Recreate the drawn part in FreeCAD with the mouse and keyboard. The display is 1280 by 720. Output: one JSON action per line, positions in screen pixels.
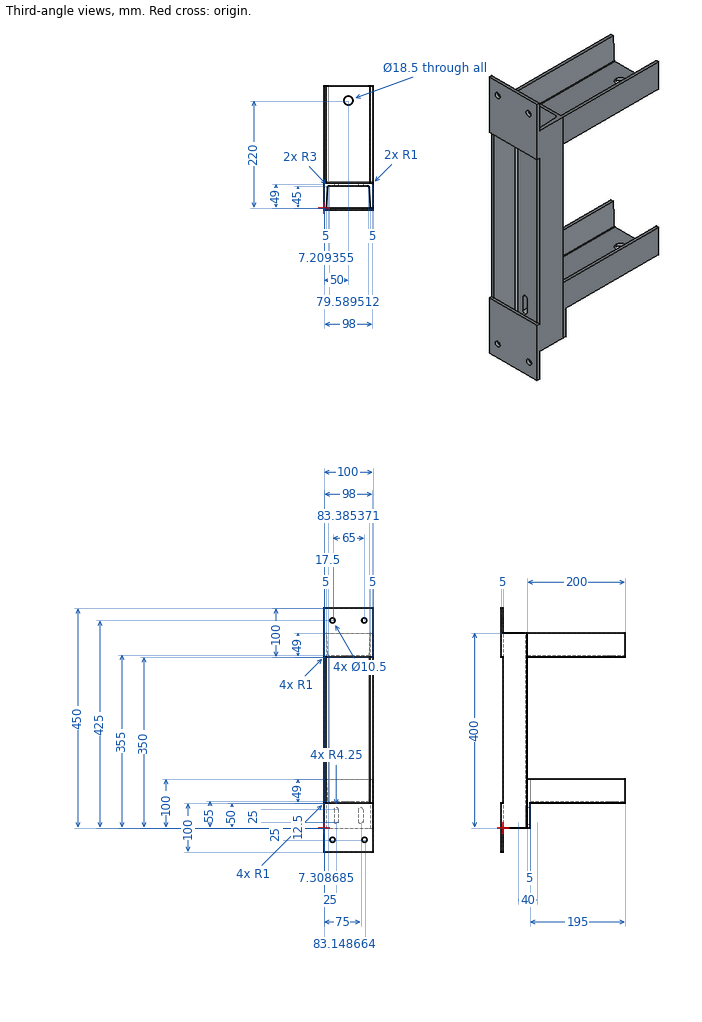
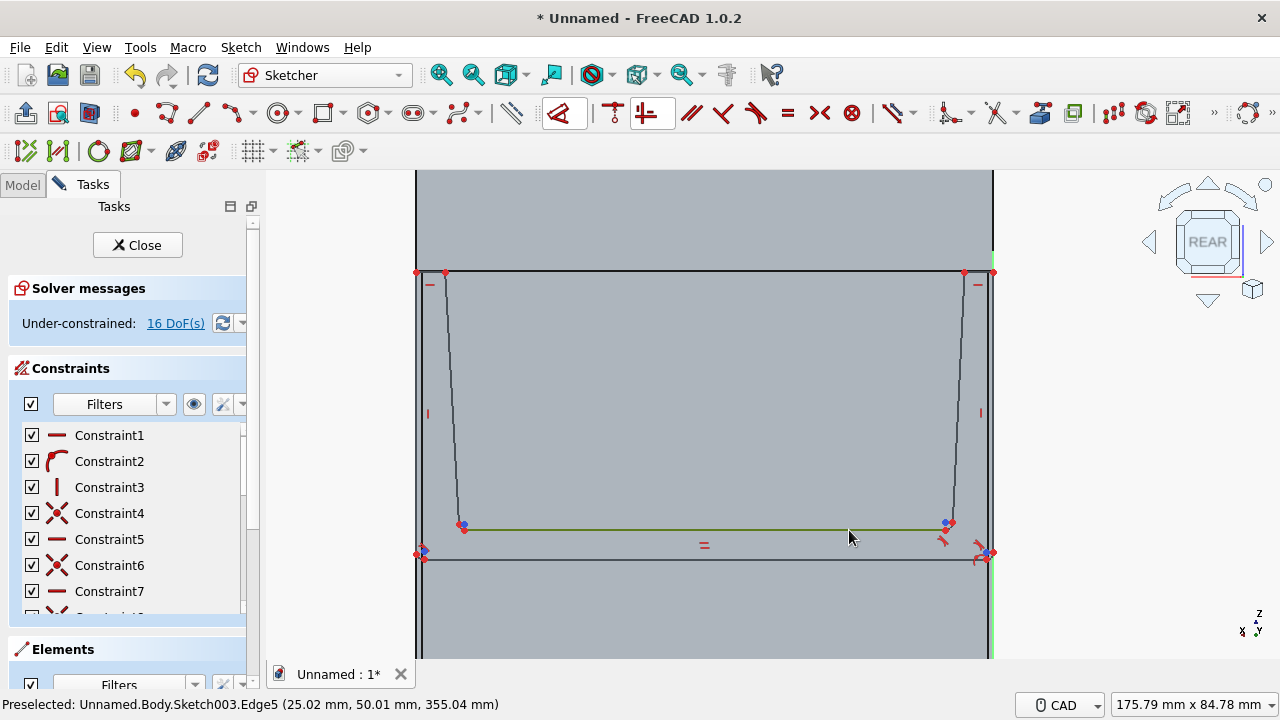
{"action": "scroll", "coordinate": [461, 528], "scroll_direction": "up", "scroll_amount": 7}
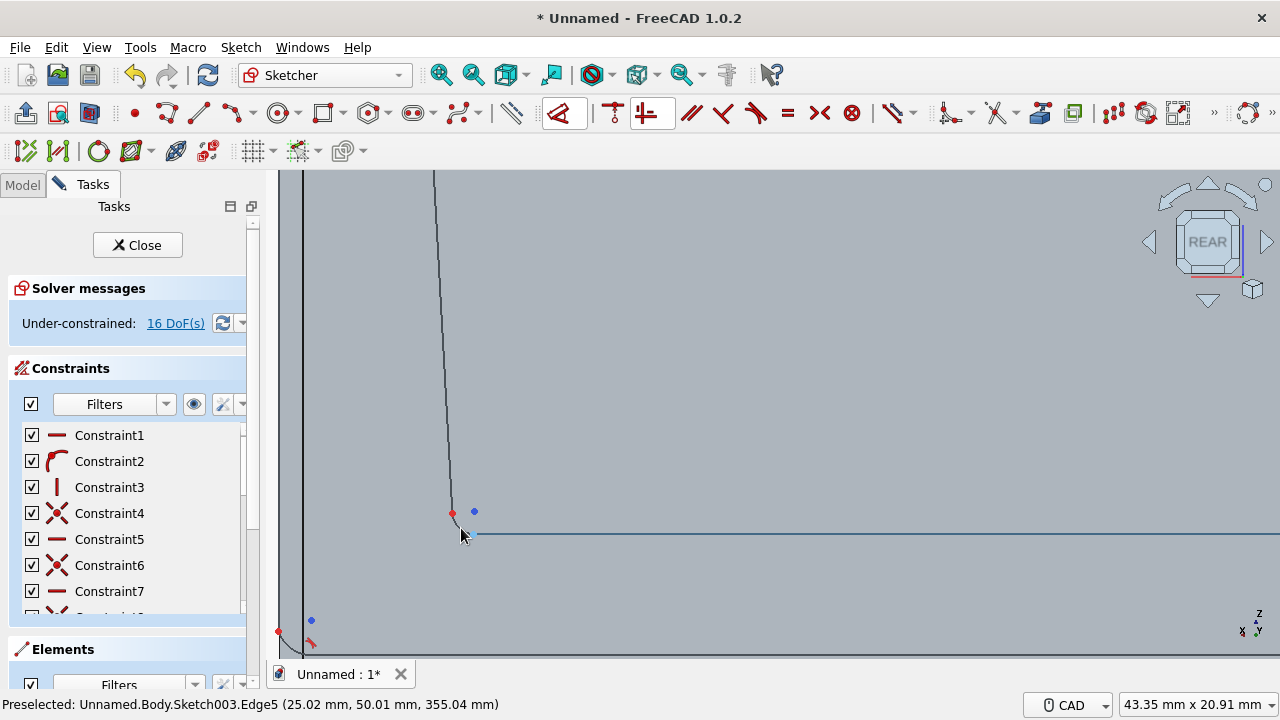
{"action": "left_click", "coordinate": [459, 528]}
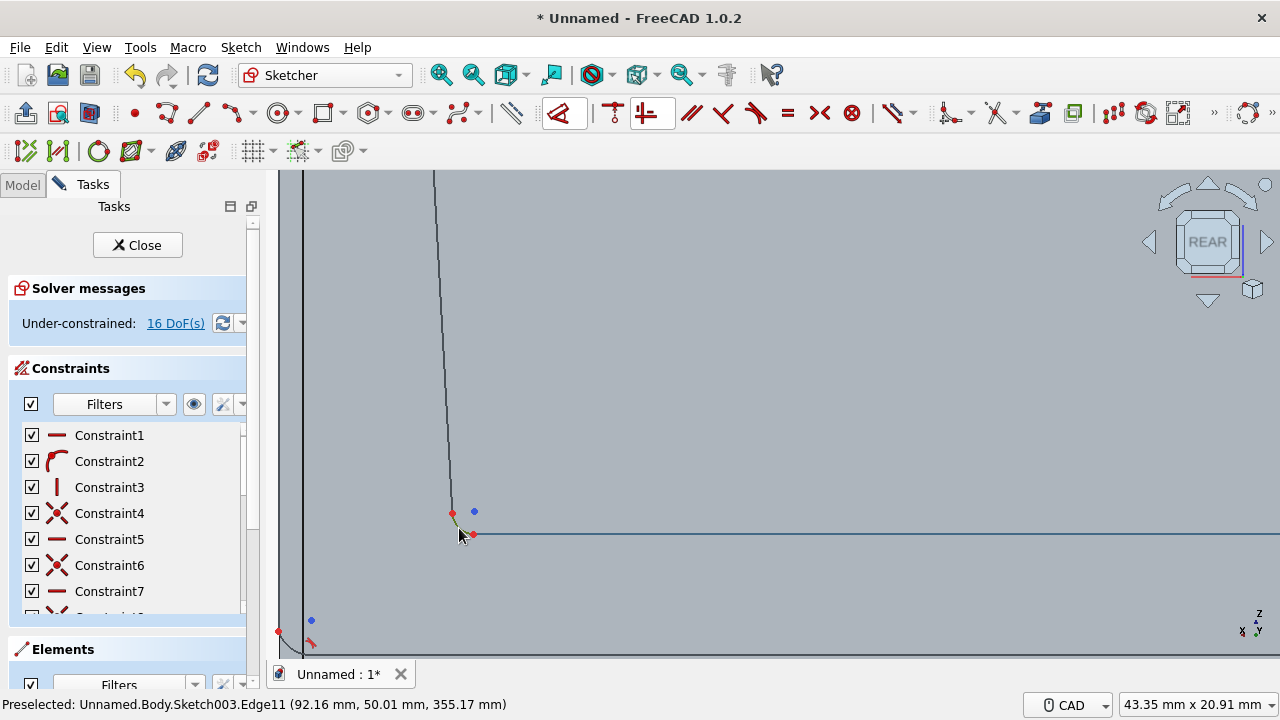
{"action": "left_click", "coordinate": [756, 114]}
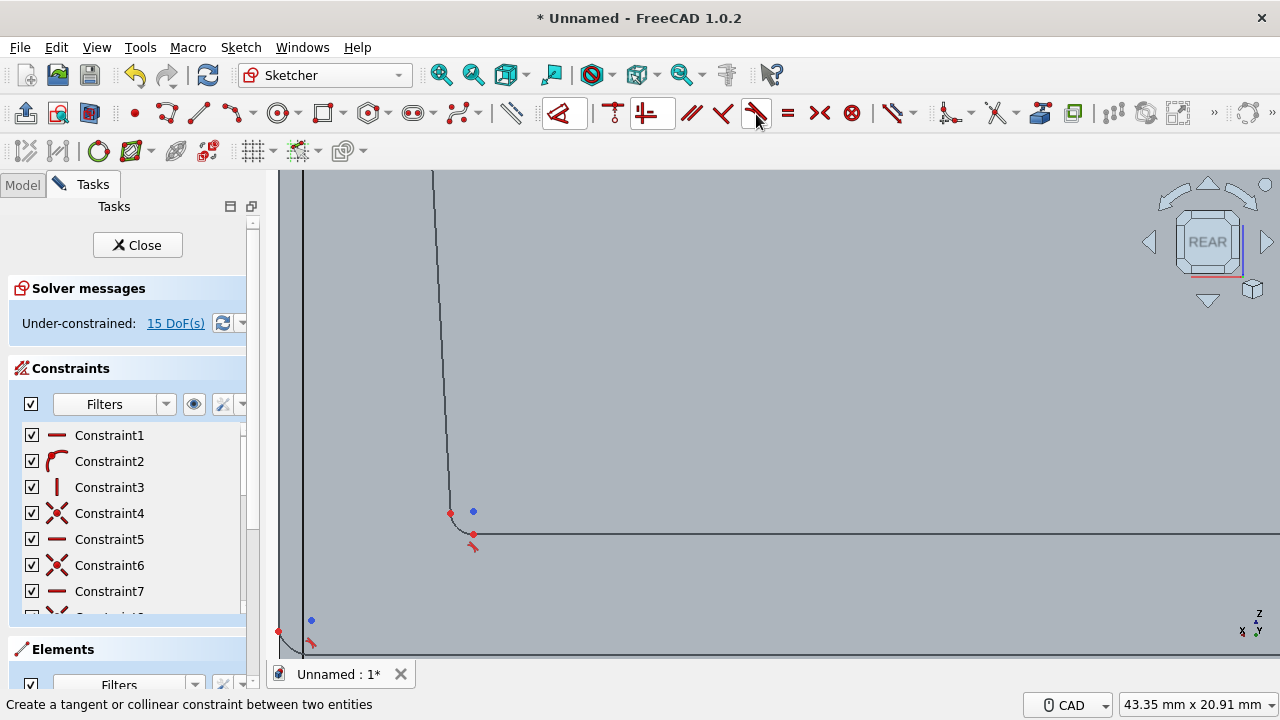
{"action": "scroll", "coordinate": [461, 528], "scroll_direction": "down", "scroll_amount": 7}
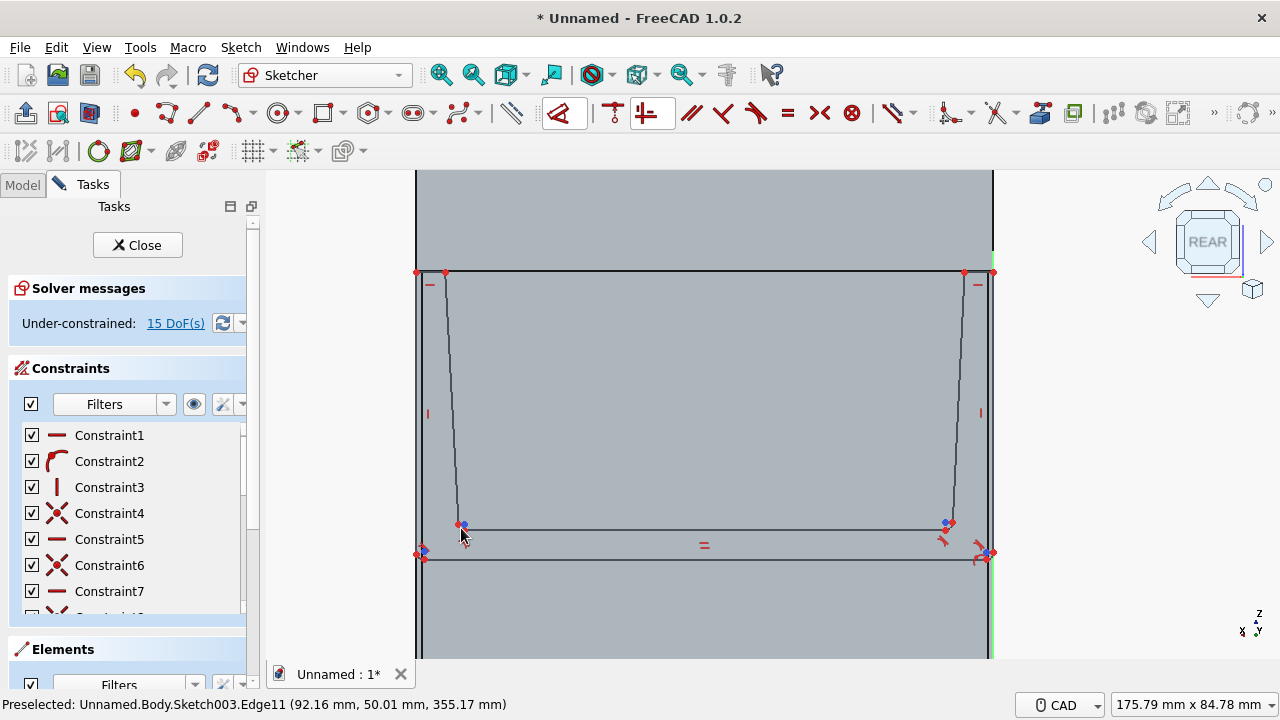
{"action": "left_click", "coordinate": [455, 449]}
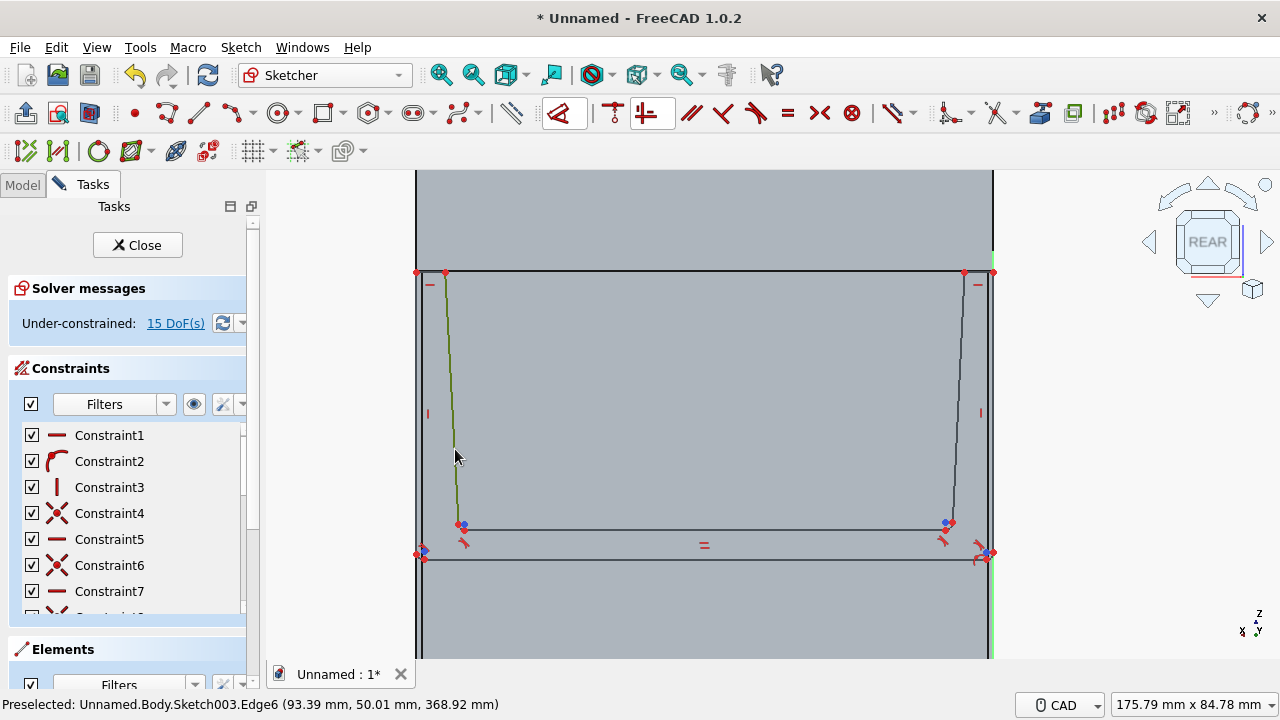
{"action": "scroll", "coordinate": [460, 529], "scroll_direction": "up", "scroll_amount": 7}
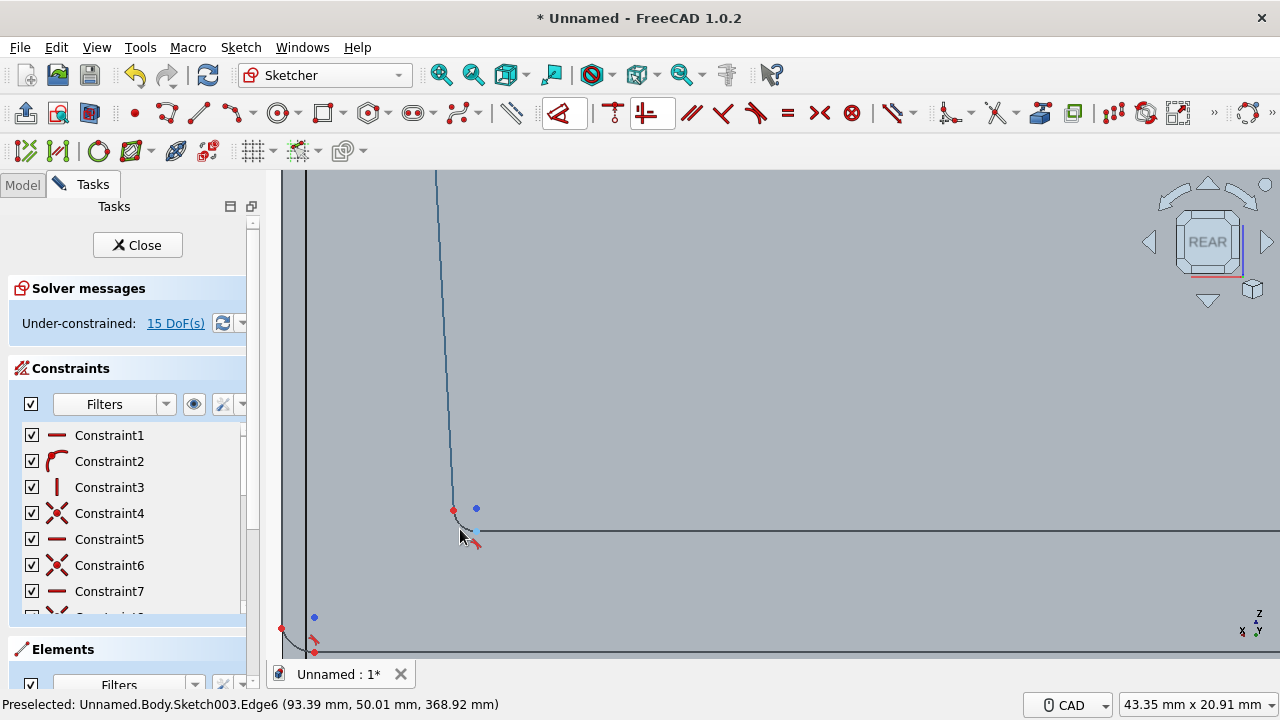
{"action": "left_click", "coordinate": [461, 525]}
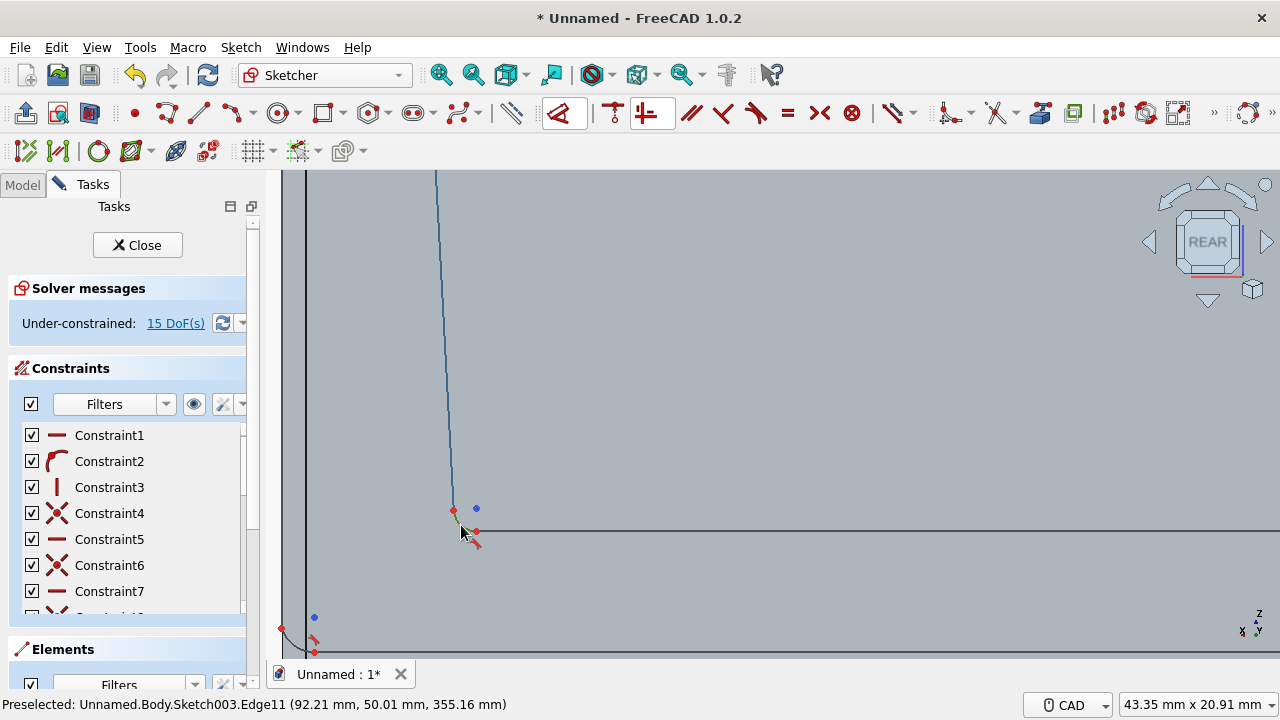
{"action": "left_click", "coordinate": [756, 114]}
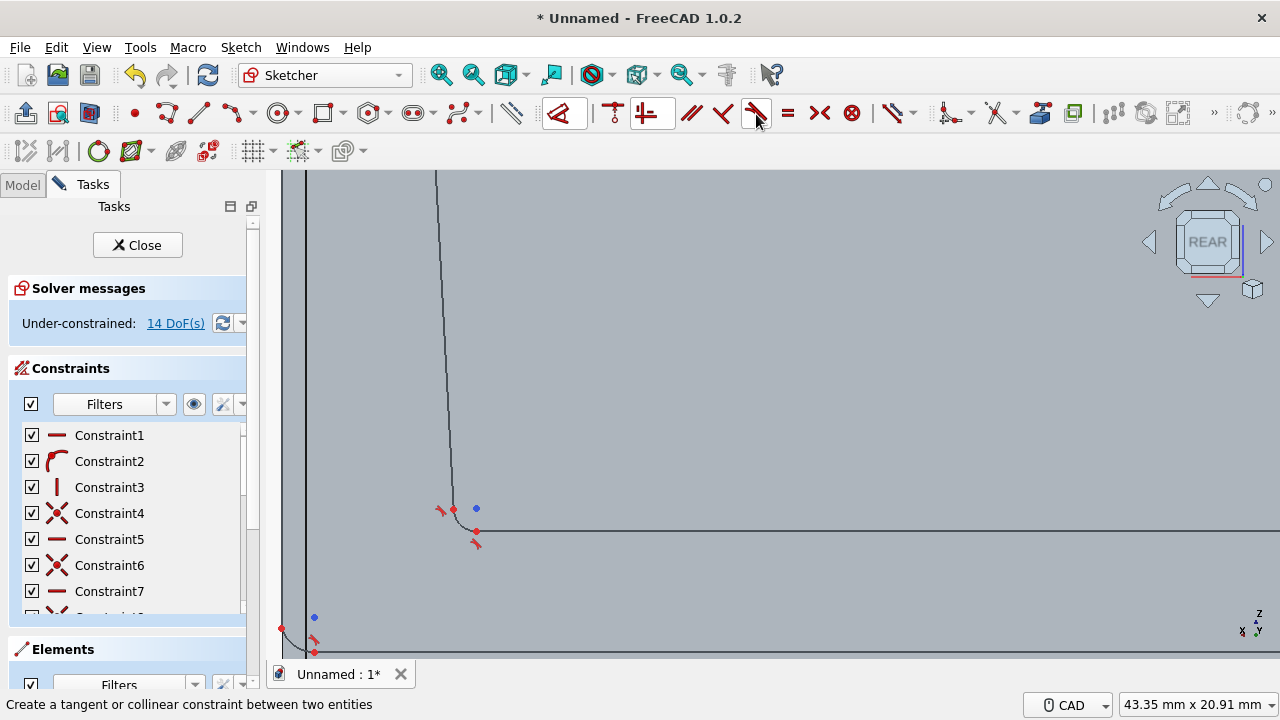
{"action": "scroll", "coordinate": [460, 529], "scroll_direction": "down", "scroll_amount": 7}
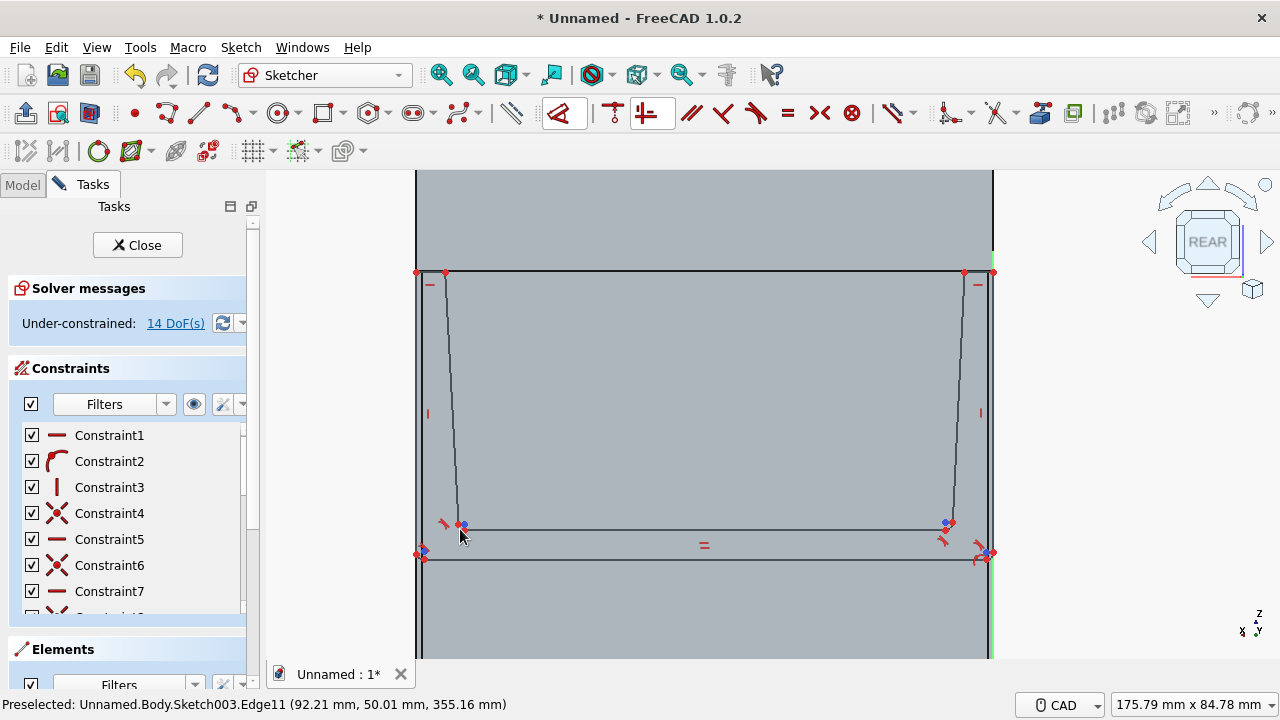
{"action": "left_click", "coordinate": [416, 357]}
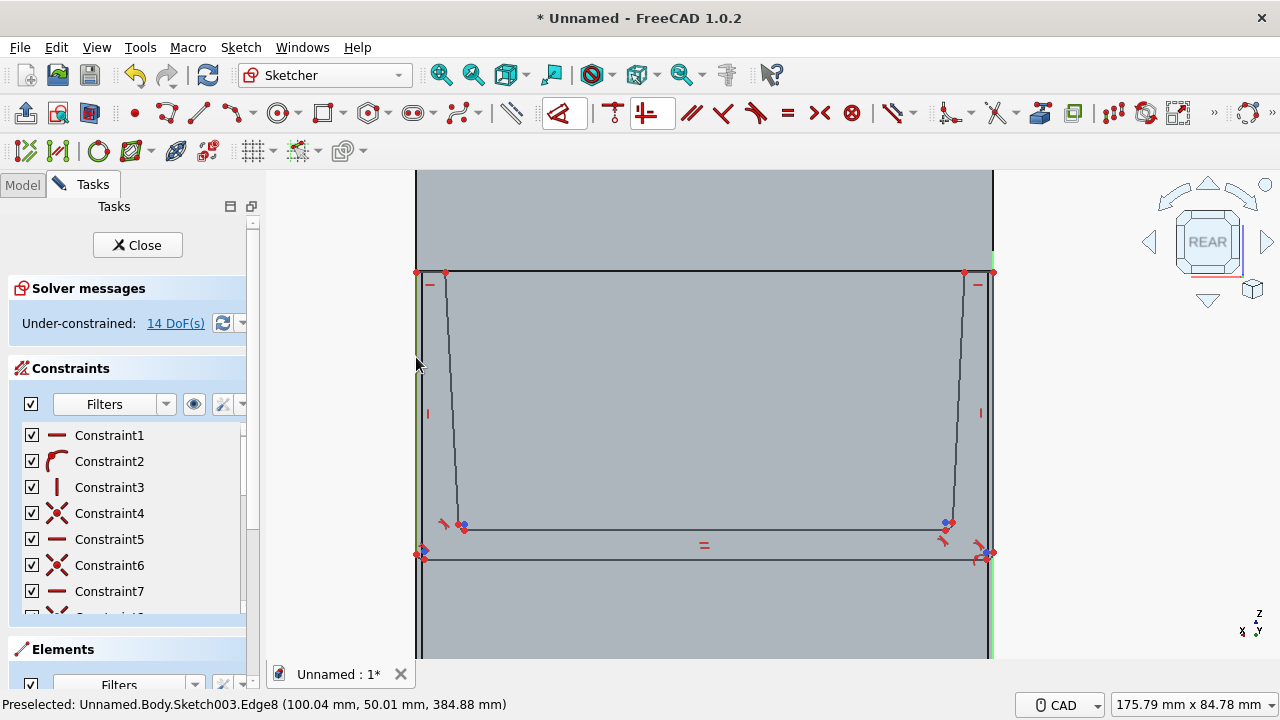
{"action": "scroll", "coordinate": [419, 558], "scroll_direction": "up", "scroll_amount": 5}